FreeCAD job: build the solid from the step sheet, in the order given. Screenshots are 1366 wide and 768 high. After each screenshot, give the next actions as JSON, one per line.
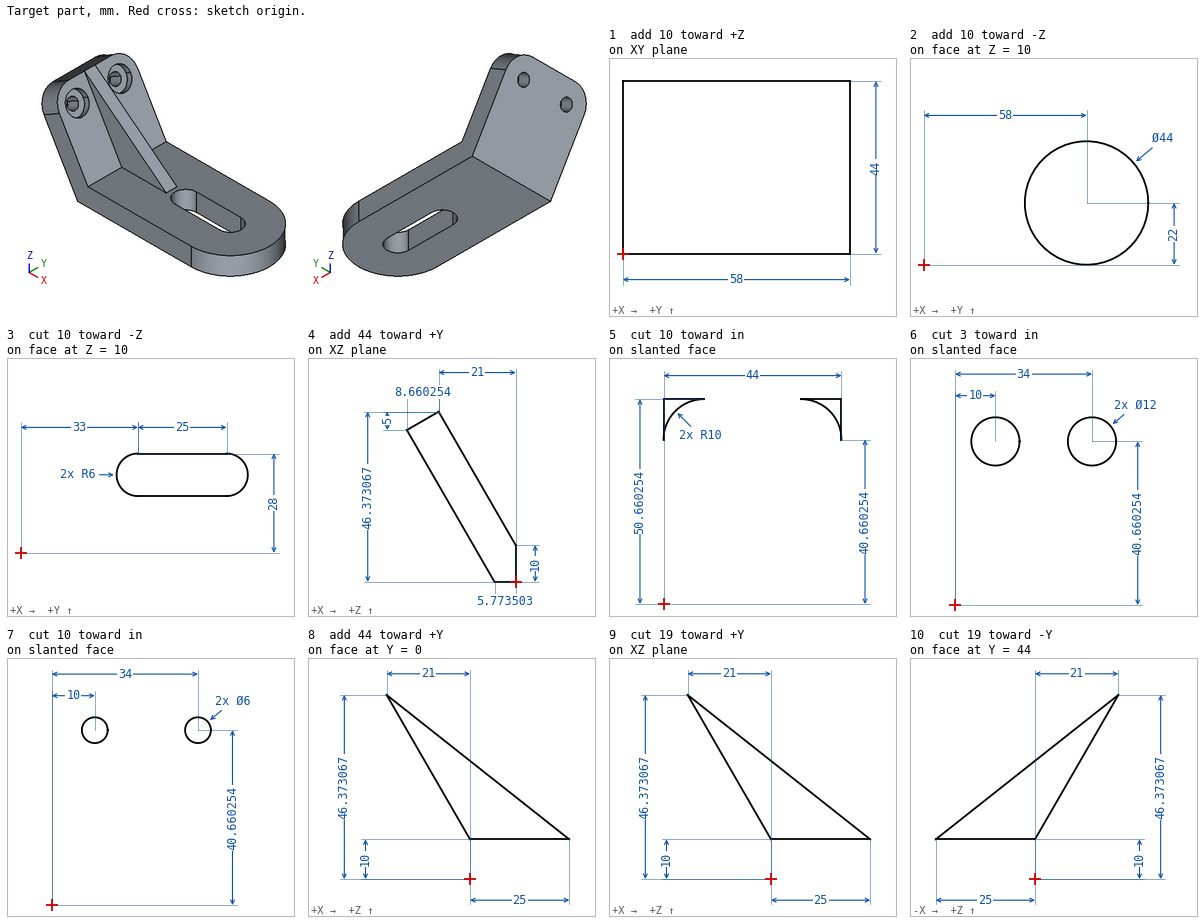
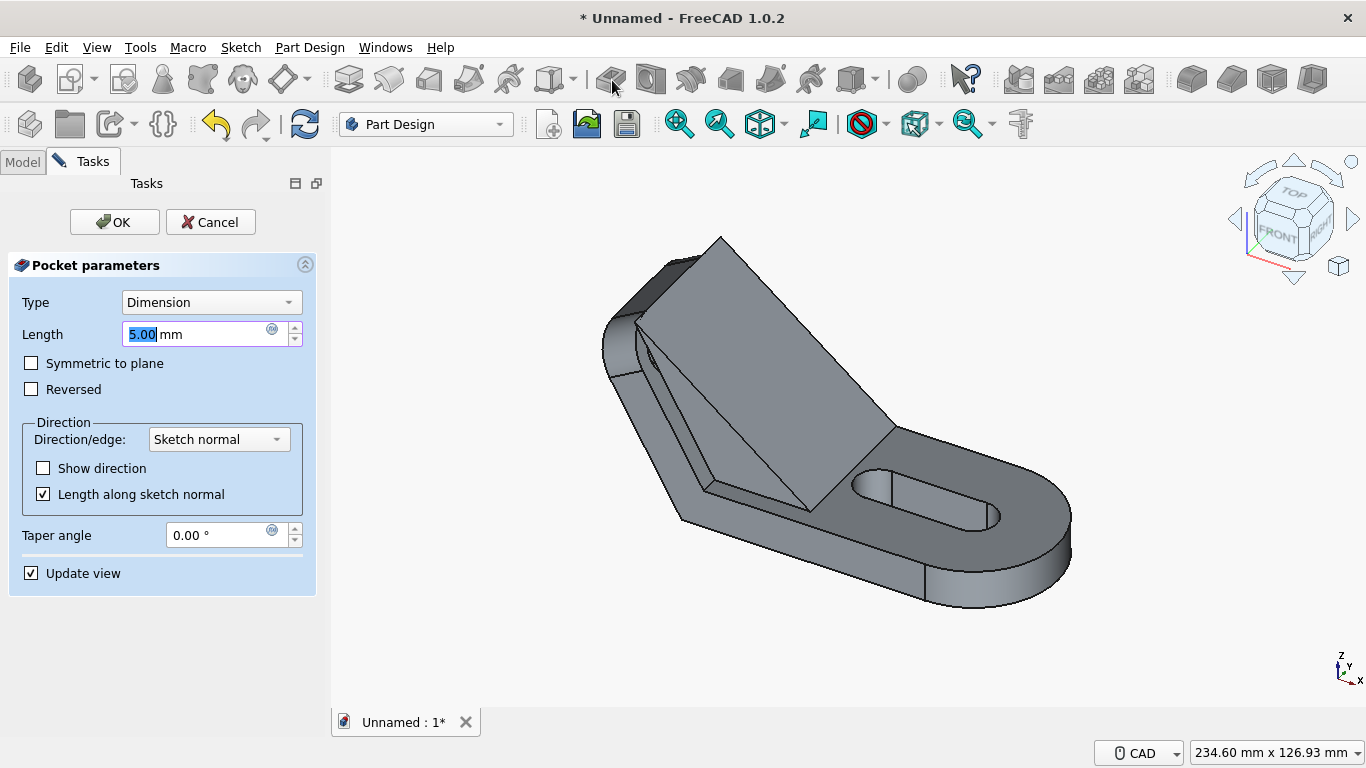
{"action": "type", "text": "19"}
{"action": "key", "text": "Tab"}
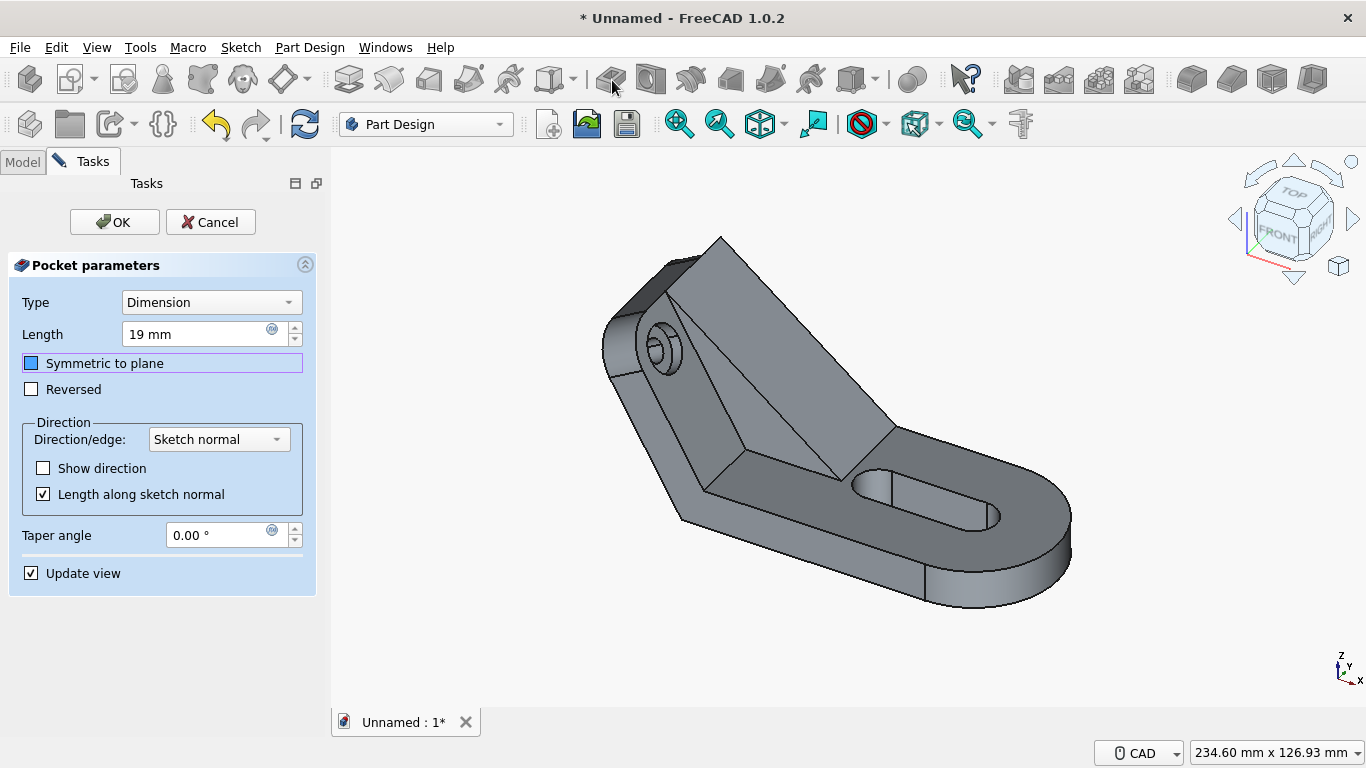
{"action": "left_click", "coordinate": [115, 222]}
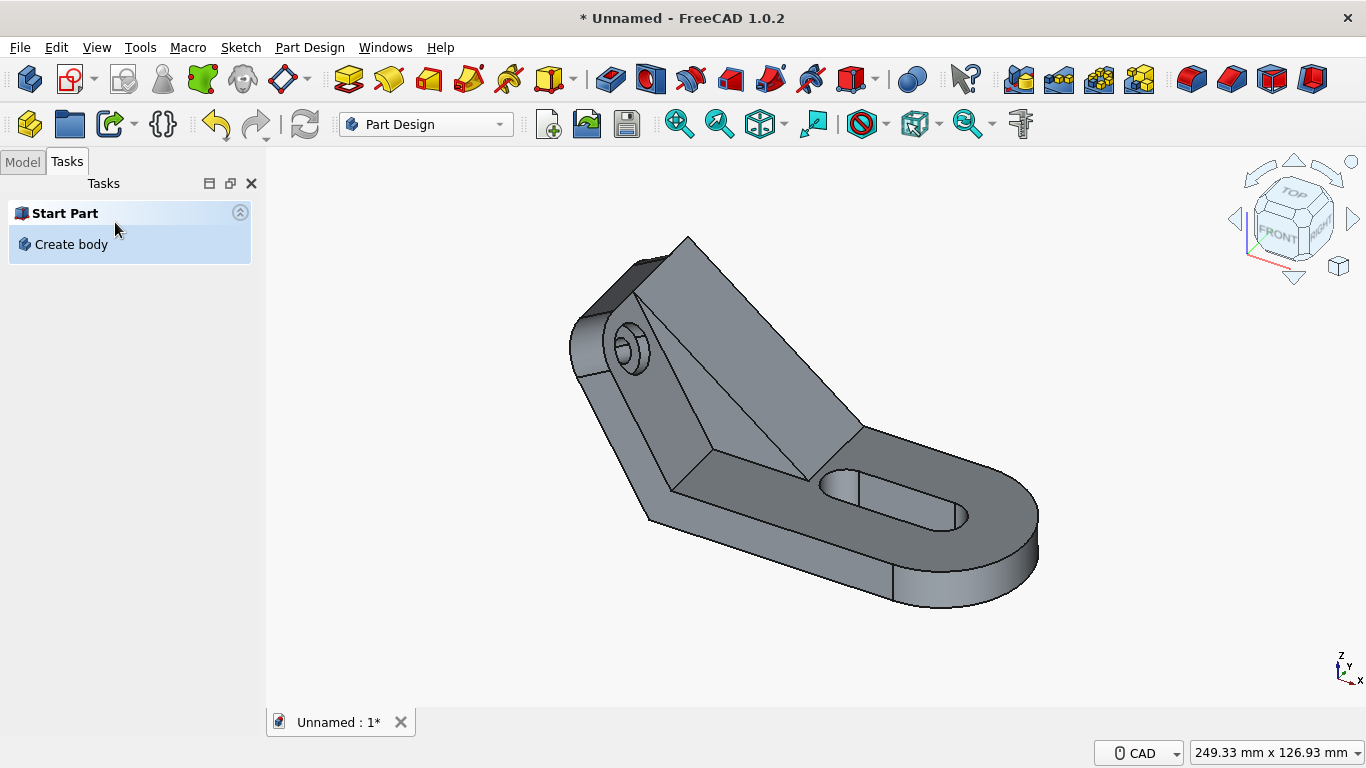
{"action": "key", "text": "4"}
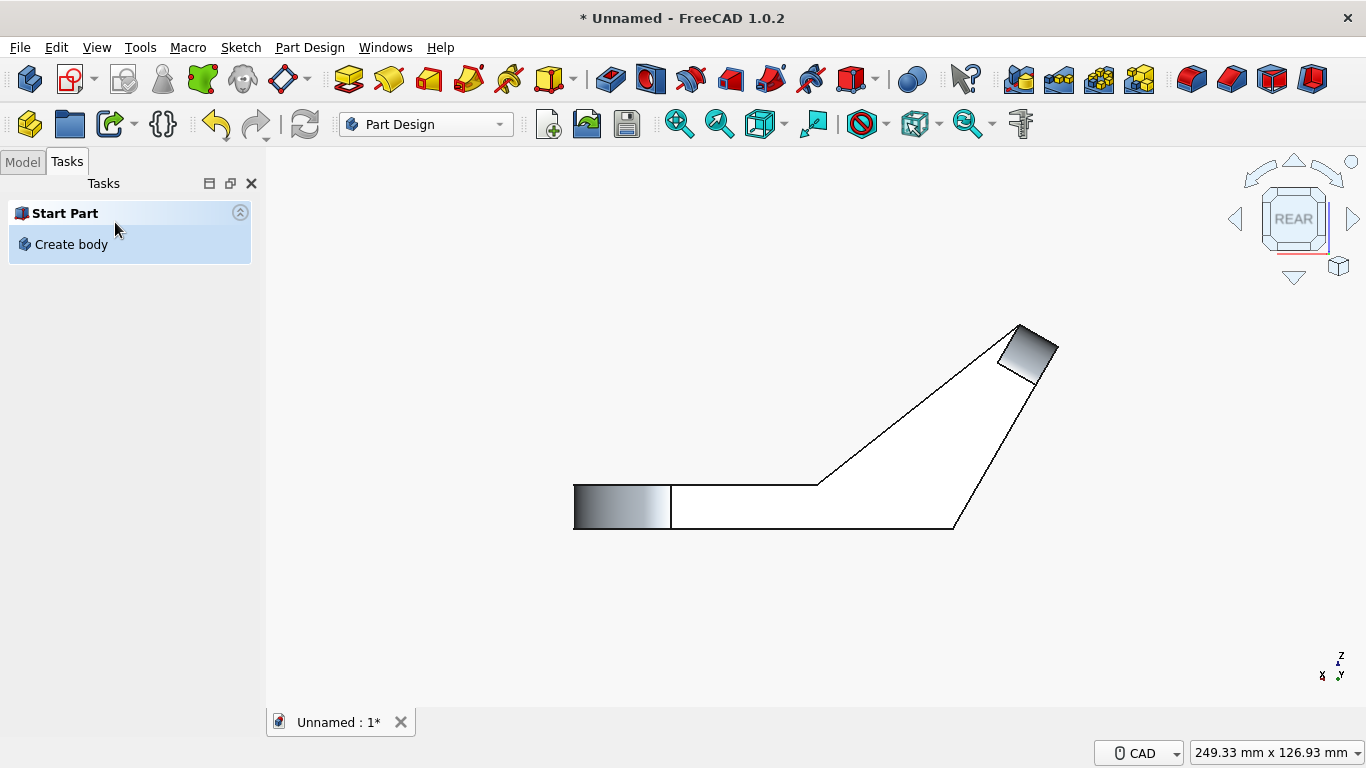
{"action": "key", "text": "v f"}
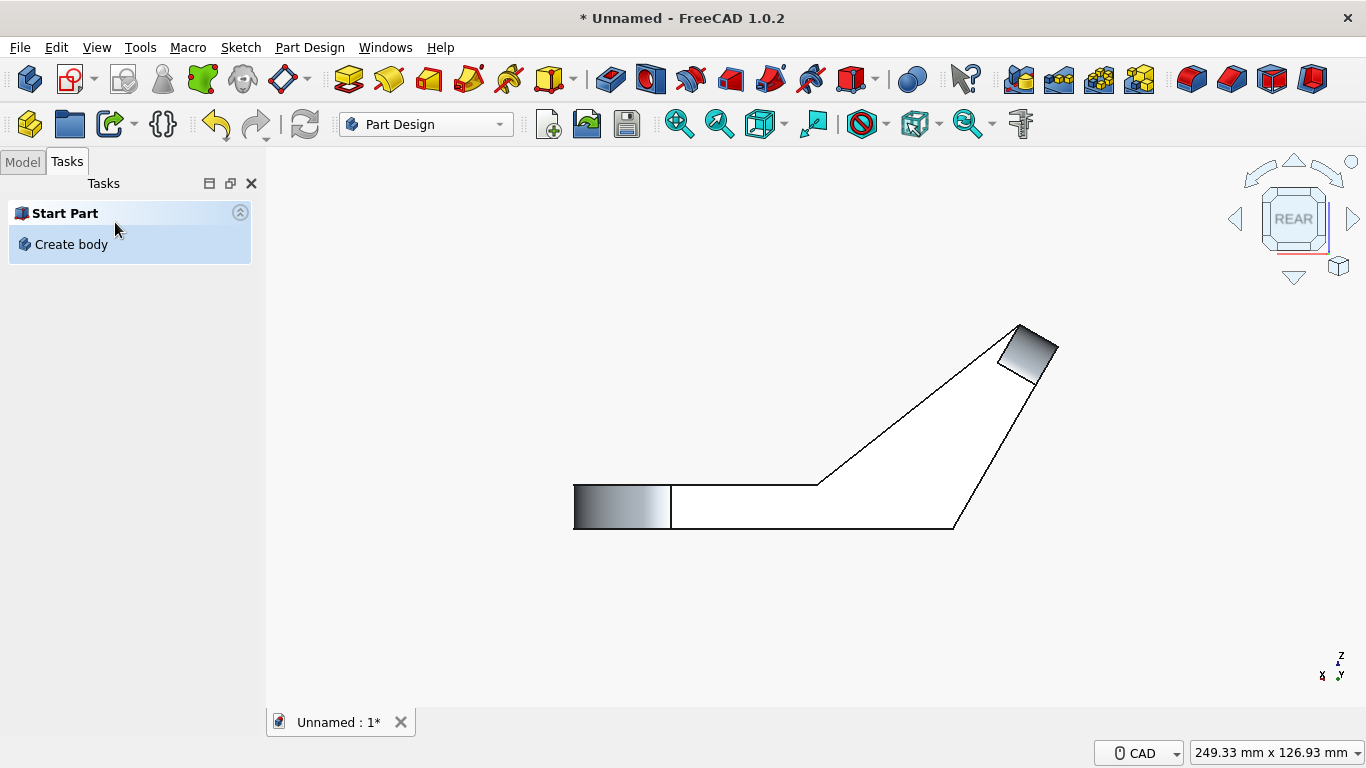
{"action": "left_click", "coordinate": [906, 484]}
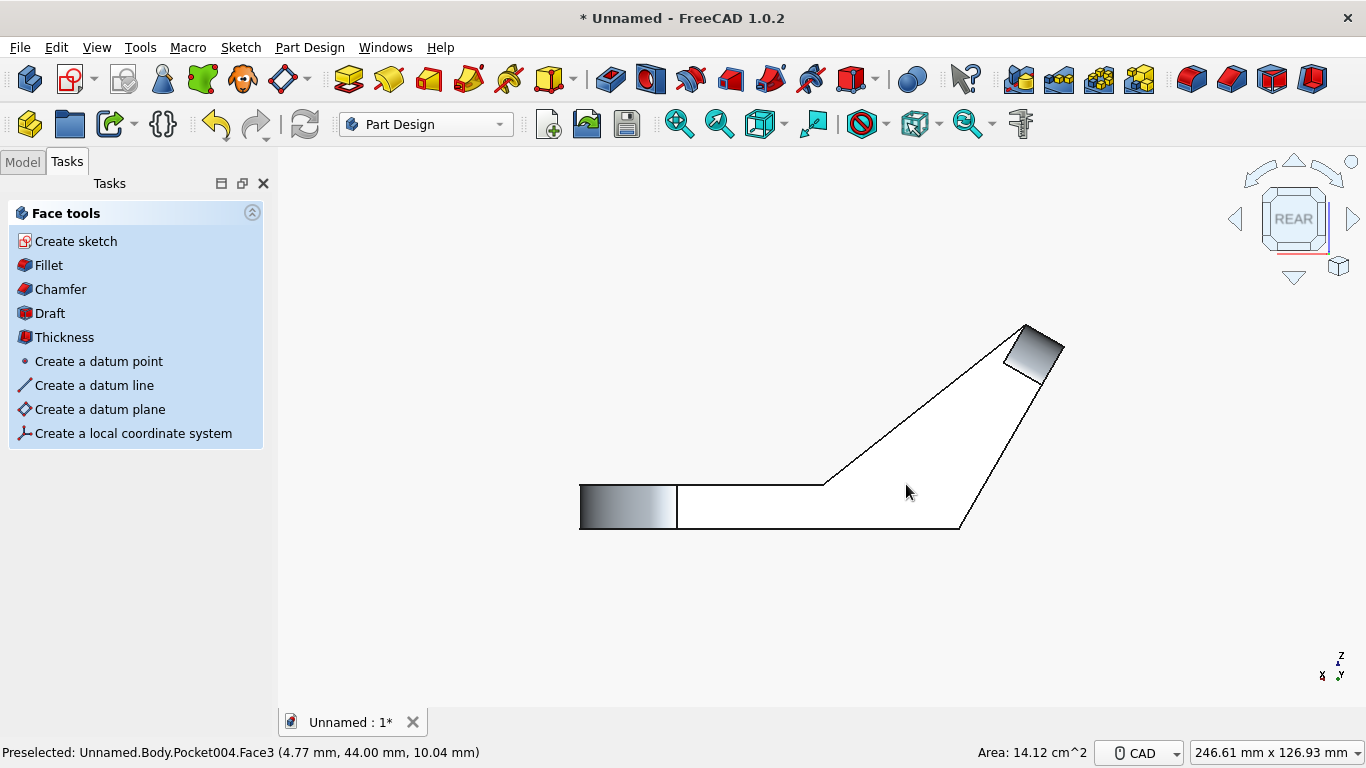
{"action": "left_click", "coordinate": [70, 80]}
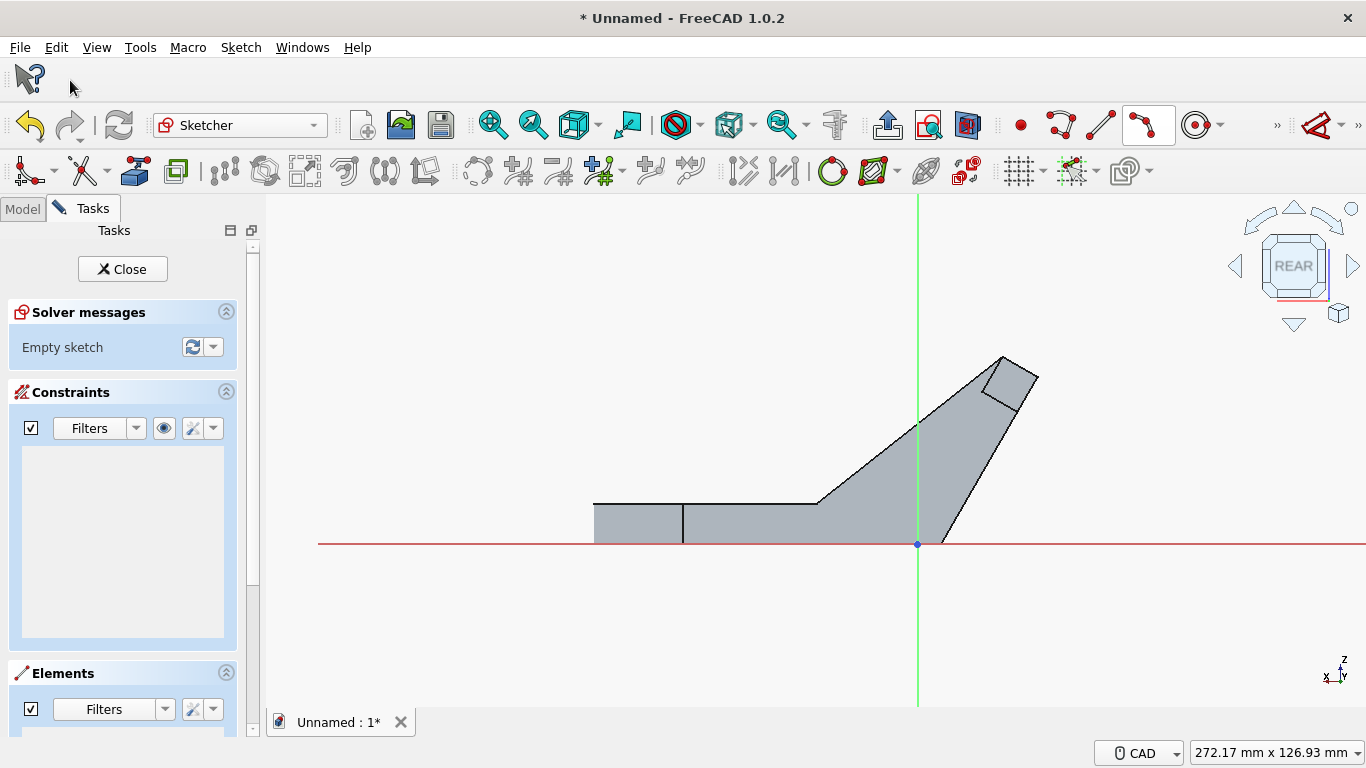
{"action": "scroll", "coordinate": [1107, 451], "scroll_direction": "up", "scroll_amount": 3}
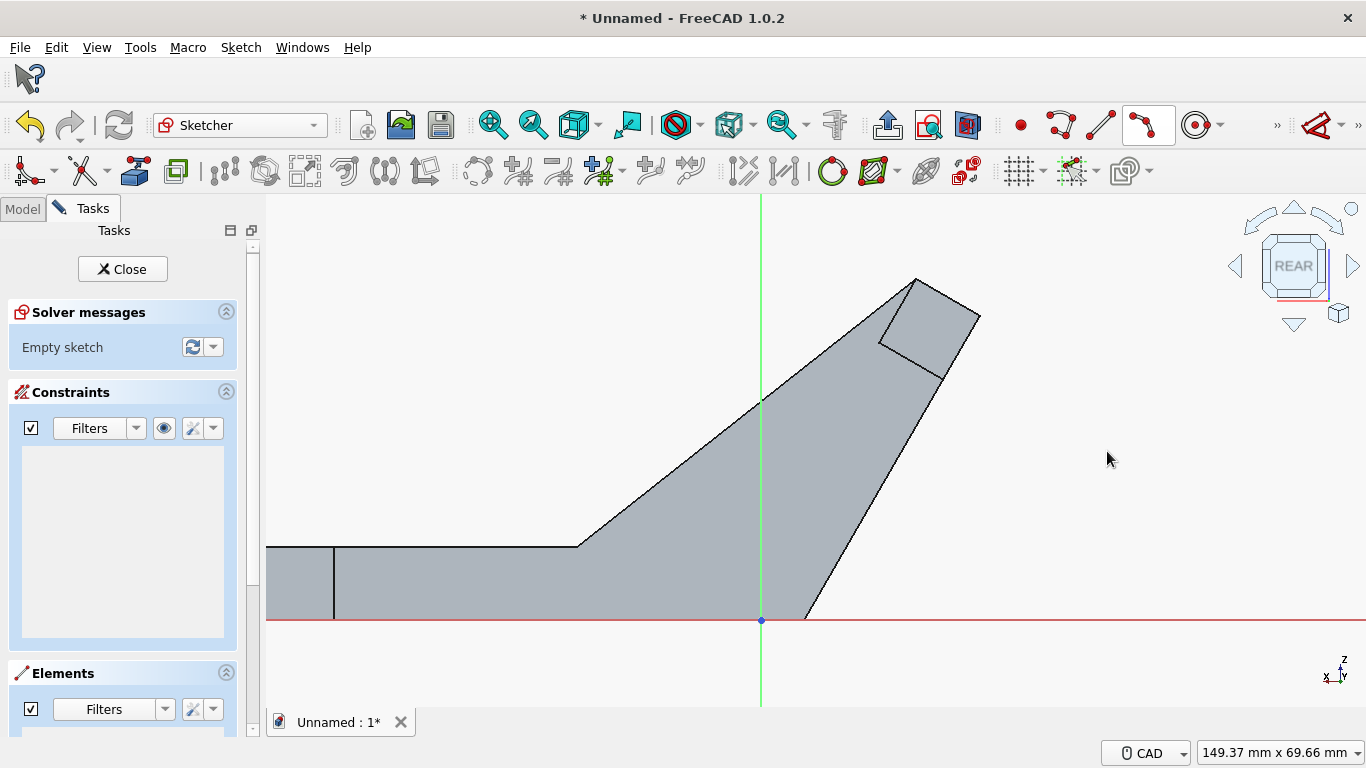
{"action": "left_click", "coordinate": [1062, 126]}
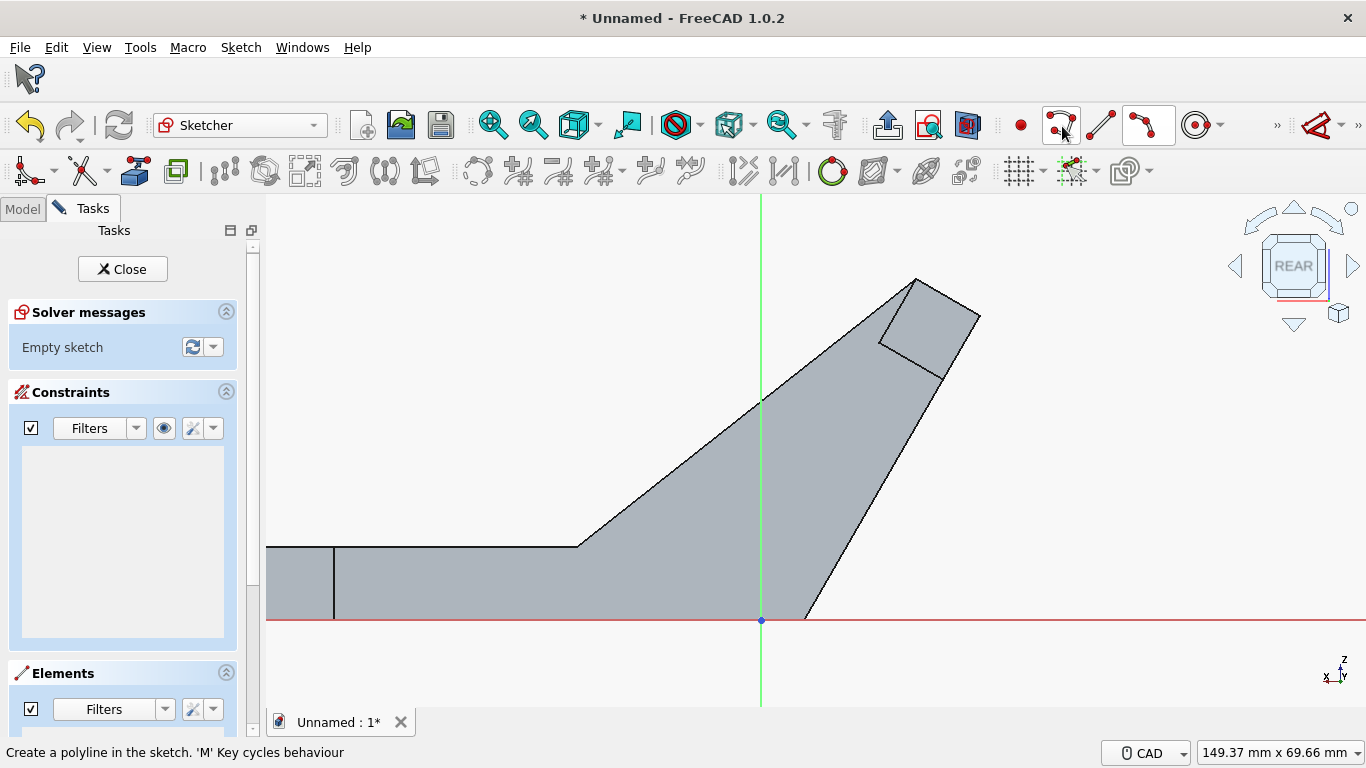
{"action": "left_click", "coordinate": [761, 547]}
{"action": "left_click", "coordinate": [916, 279]}
{"action": "left_click", "coordinate": [577, 547]}
{"action": "left_click", "coordinate": [761, 548]}
{"action": "key", "text": "Escape"}
{"action": "key", "text": "Escape"}